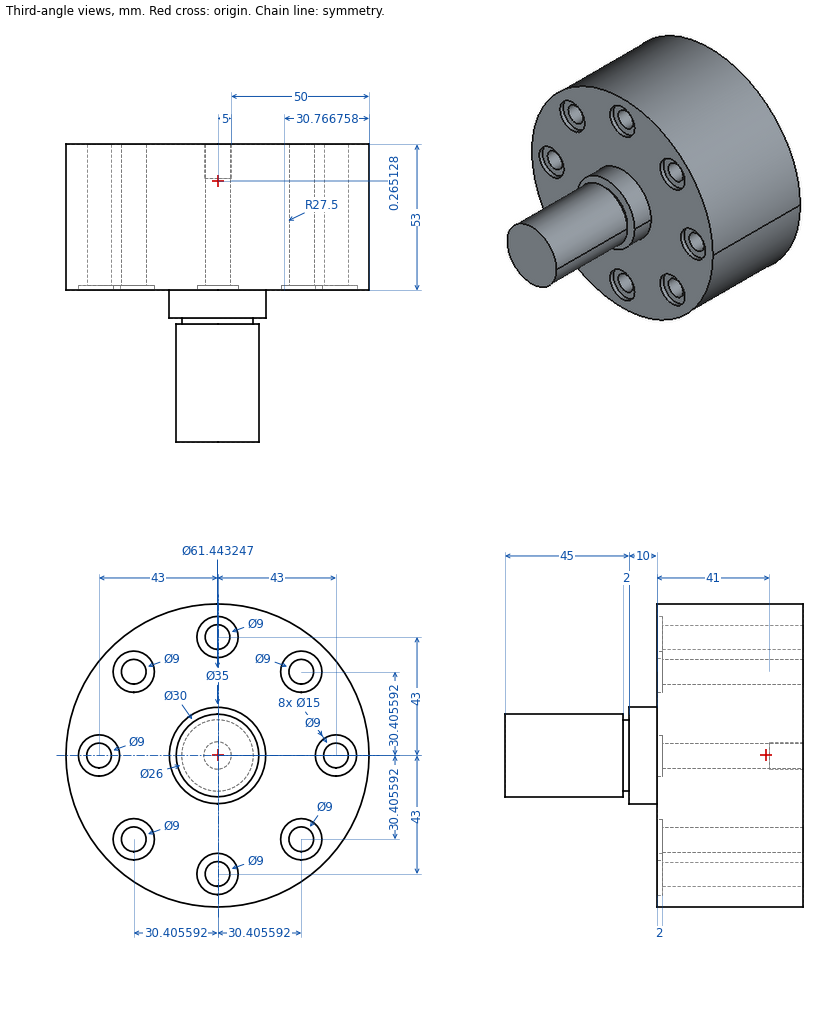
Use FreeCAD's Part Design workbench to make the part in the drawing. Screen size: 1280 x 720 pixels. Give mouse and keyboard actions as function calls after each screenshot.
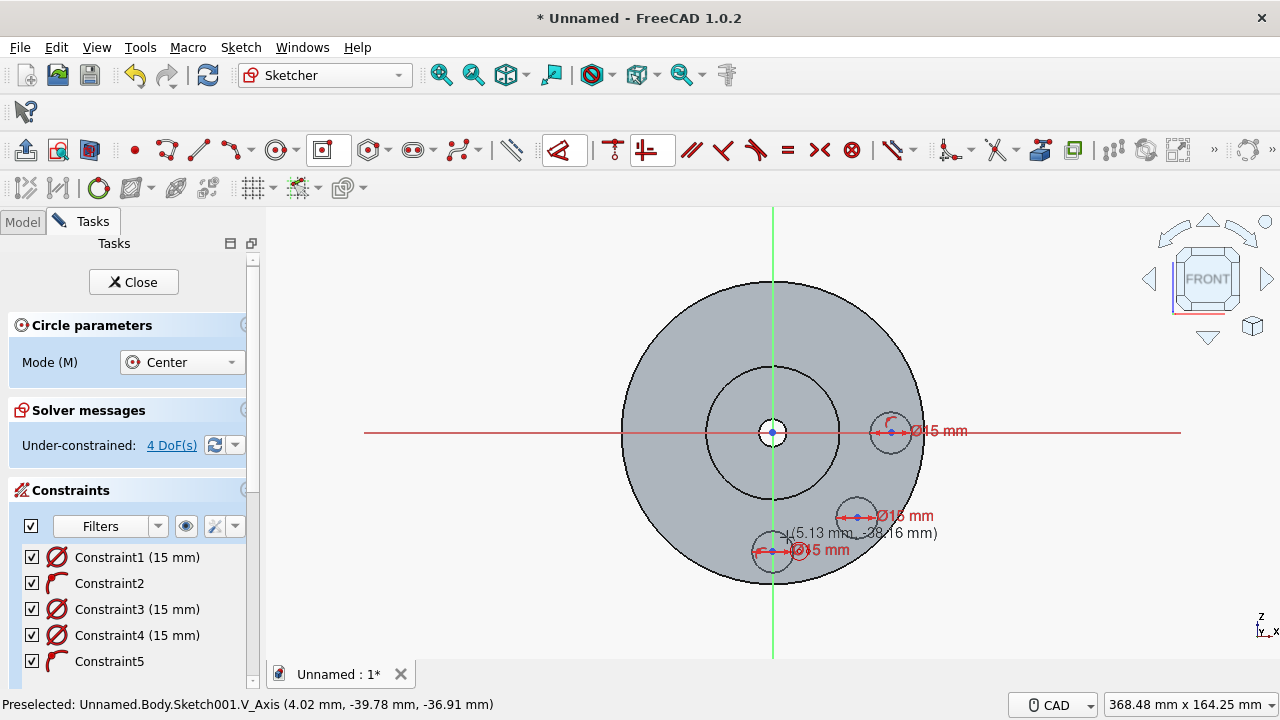
click(689, 517)
move(704, 502)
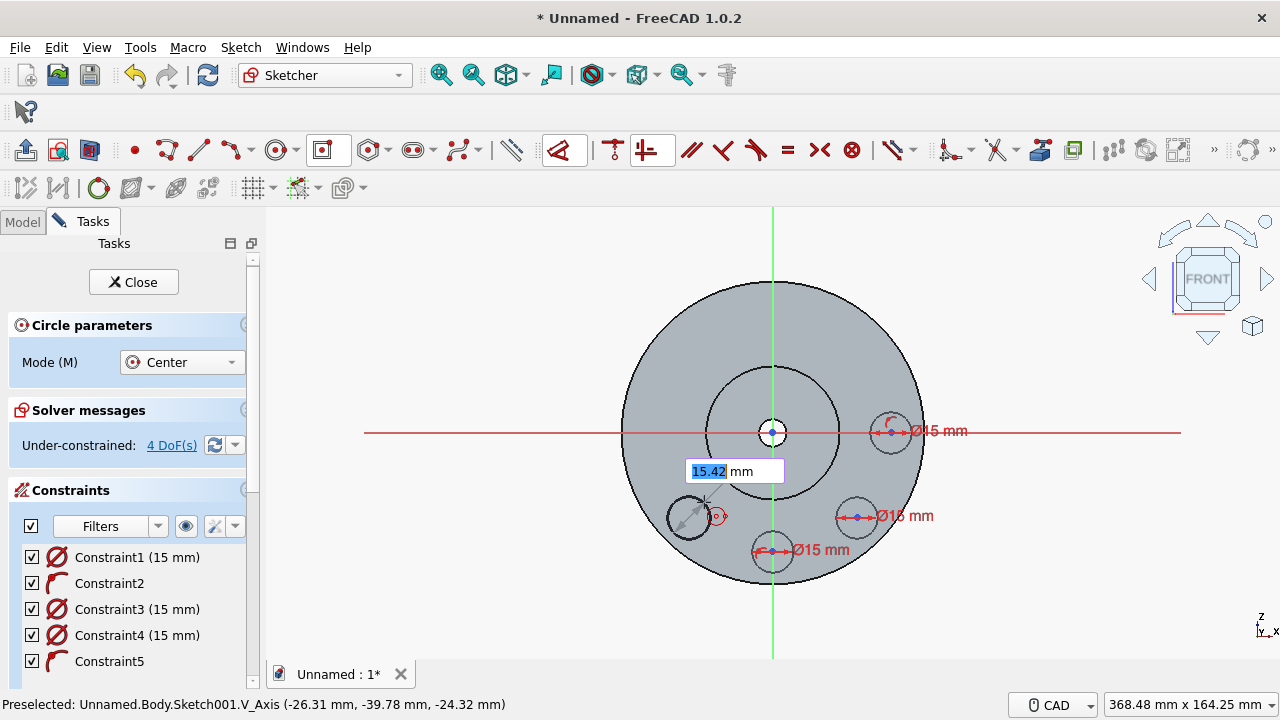
text(15)
key(Return)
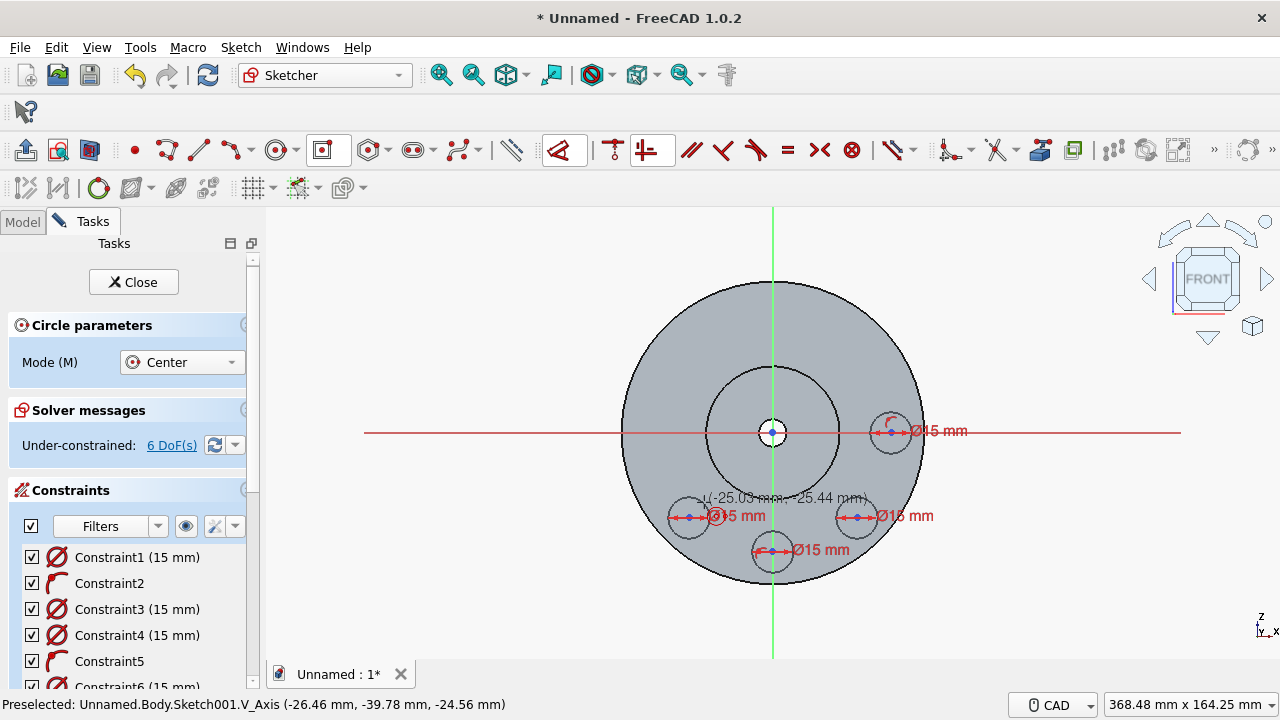
click(655, 433)
move(669, 418)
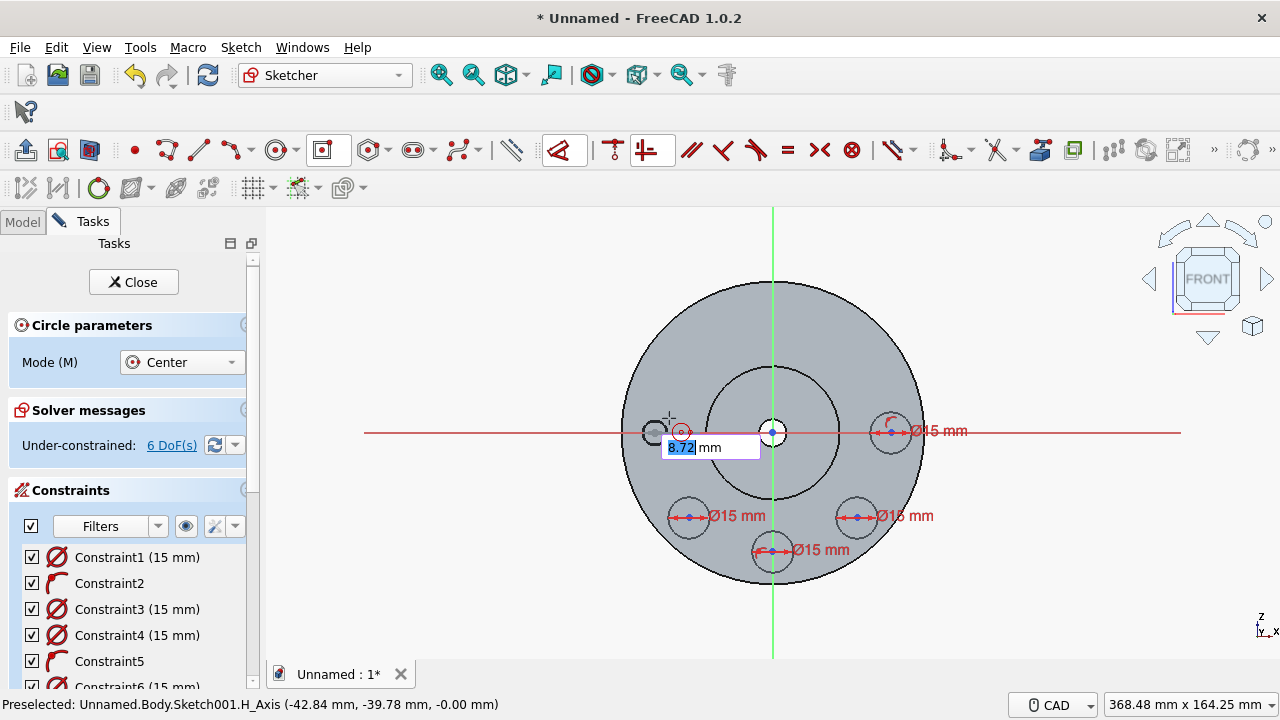
text(15)
key(Return)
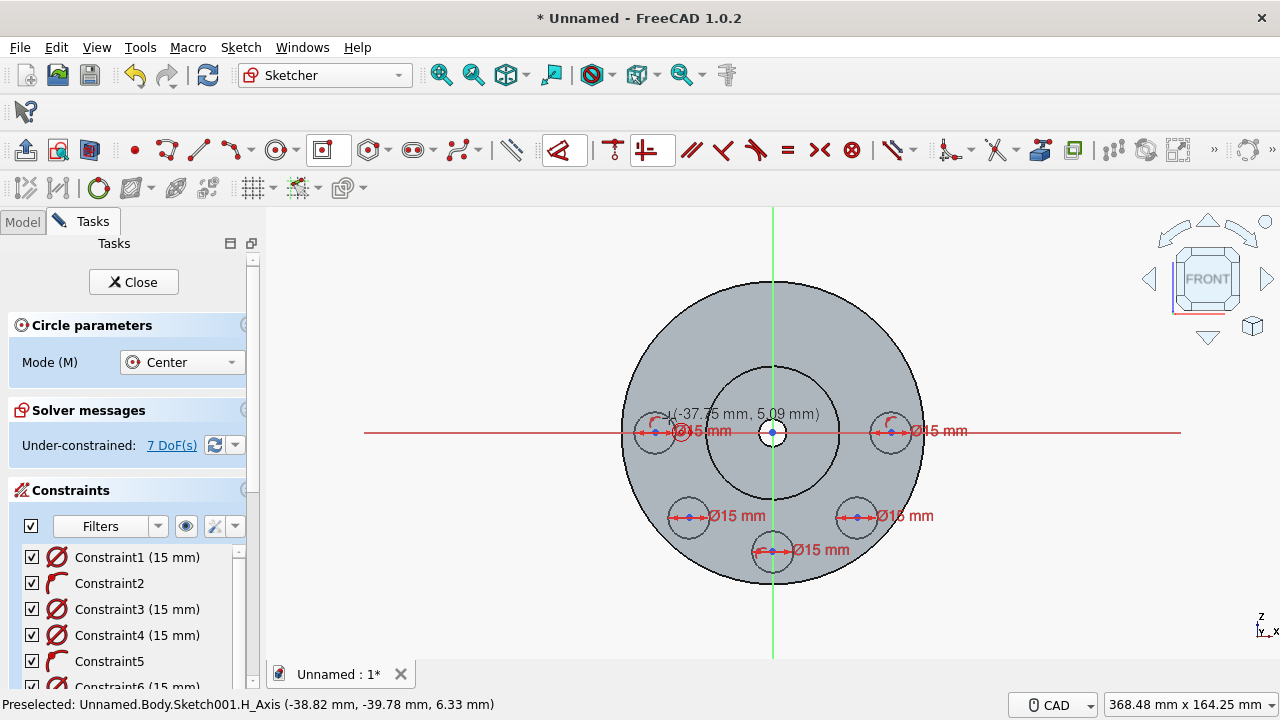
click(689, 349)
move(704, 335)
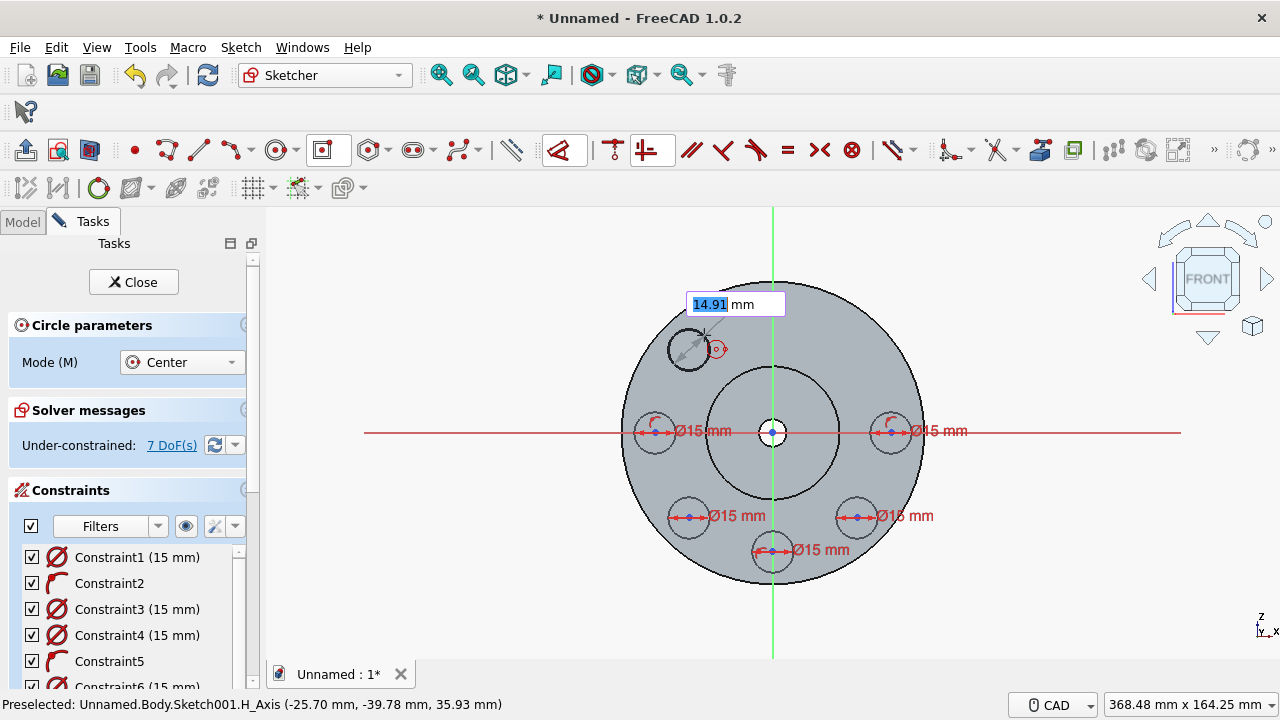
text(15)
key(Return)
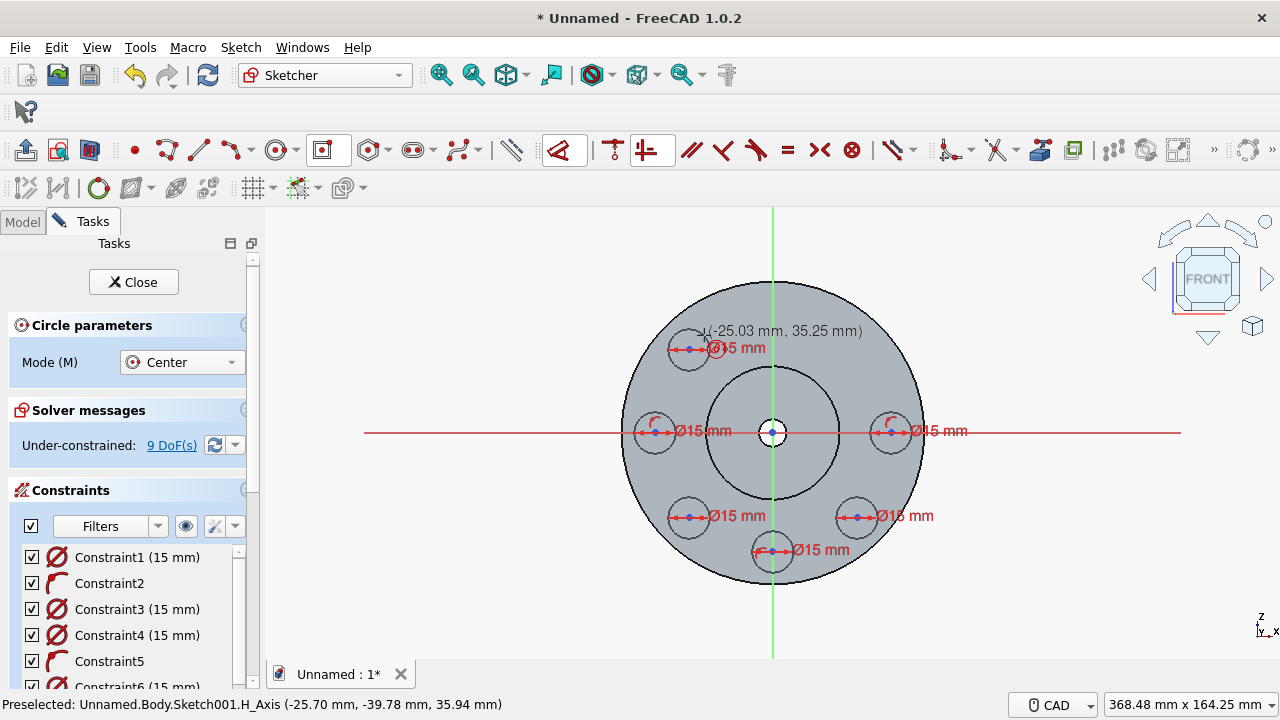
click(773, 315)
move(787, 300)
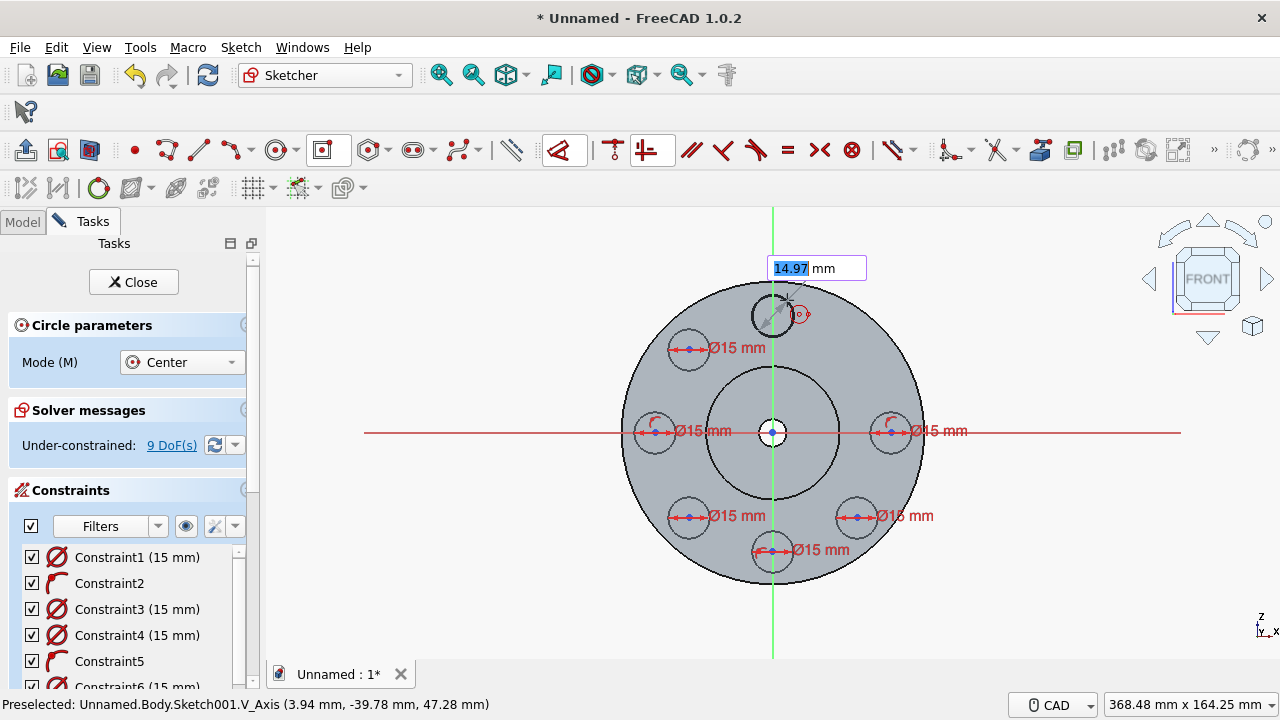
text(15)
key(Return)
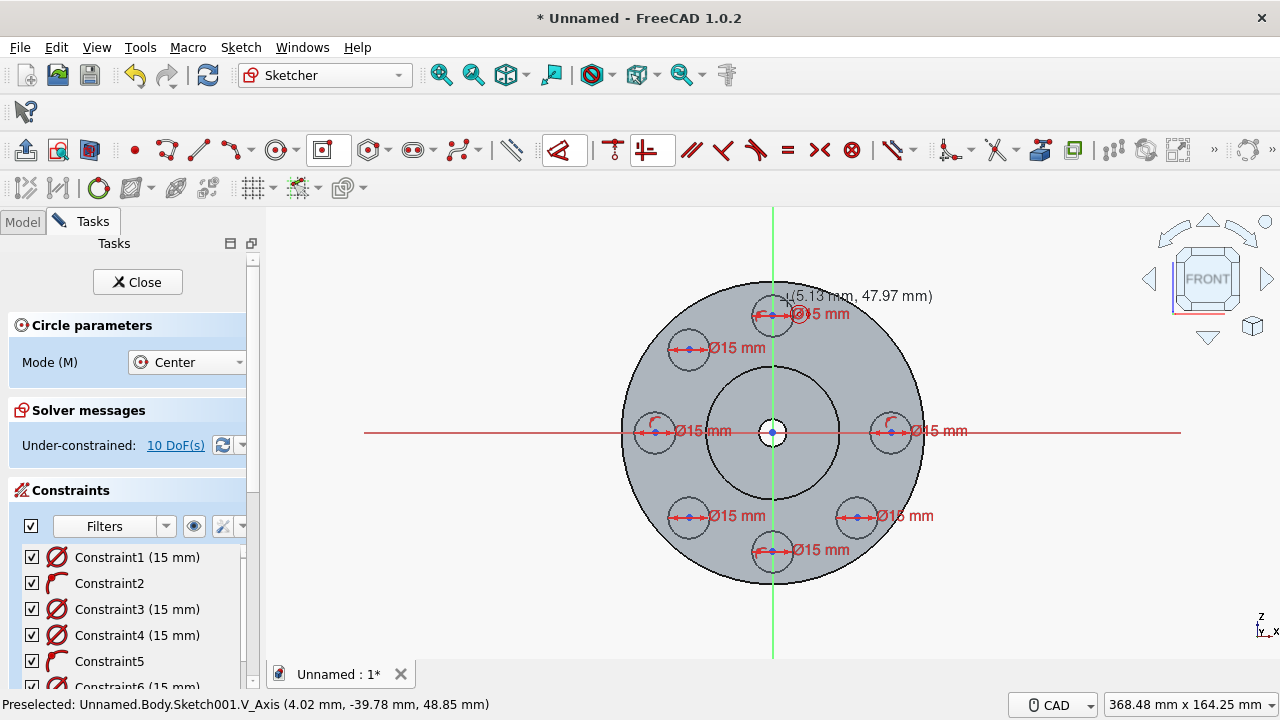
click(857, 349)
move(871, 335)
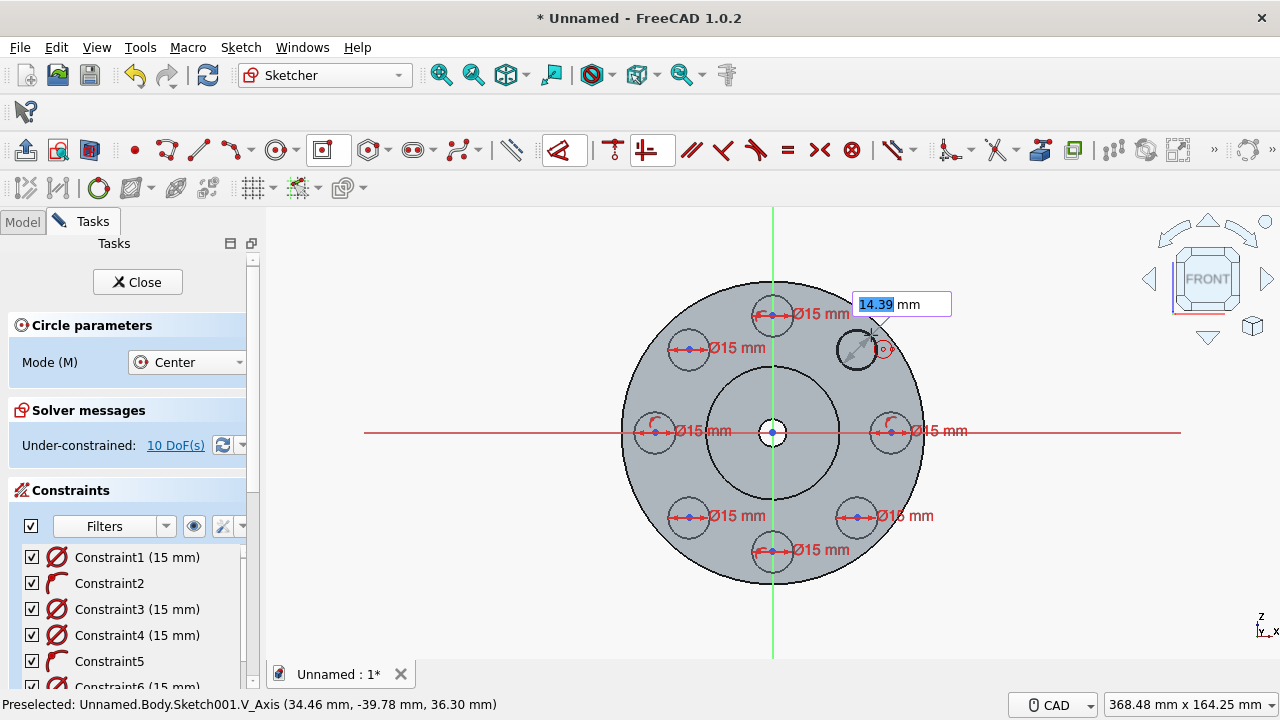
text(15)
key(Return)
key(Escape)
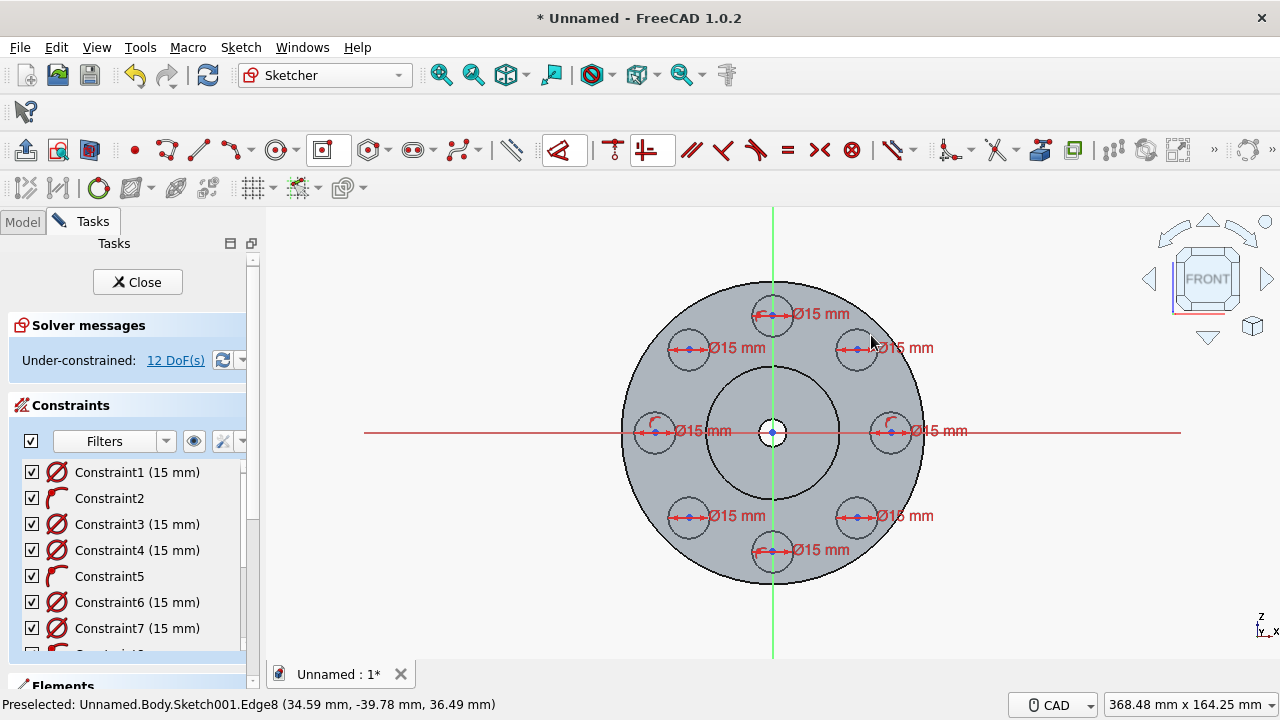
click(857, 518)